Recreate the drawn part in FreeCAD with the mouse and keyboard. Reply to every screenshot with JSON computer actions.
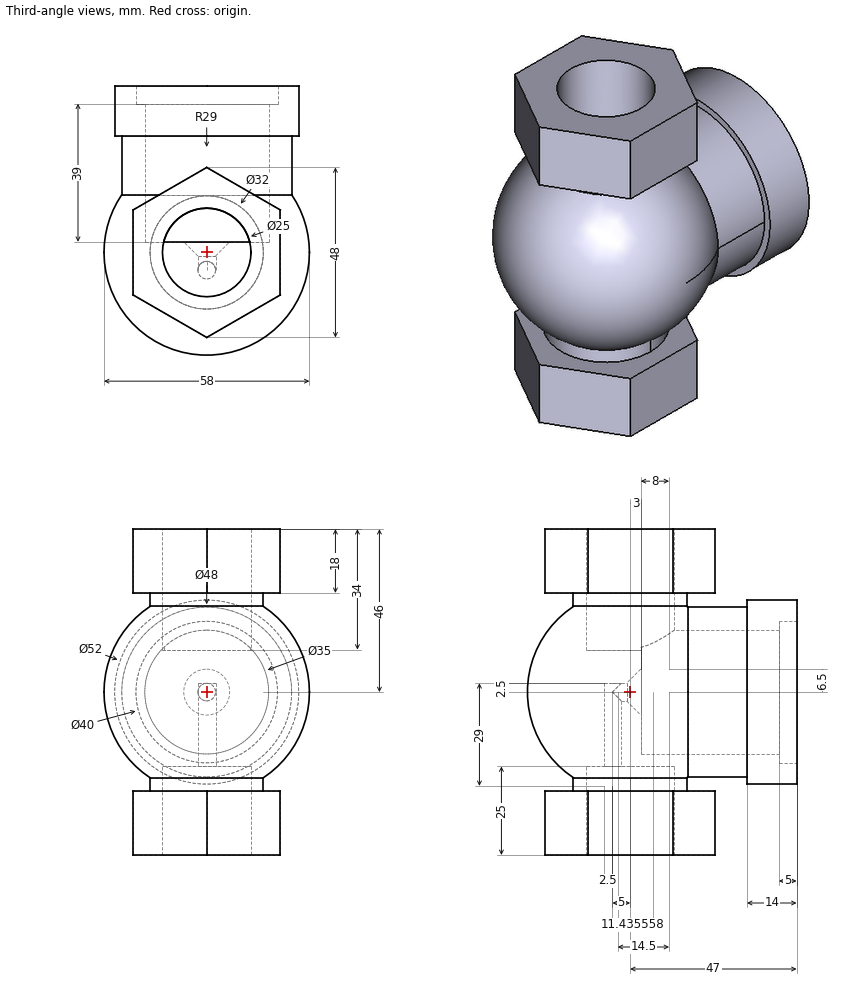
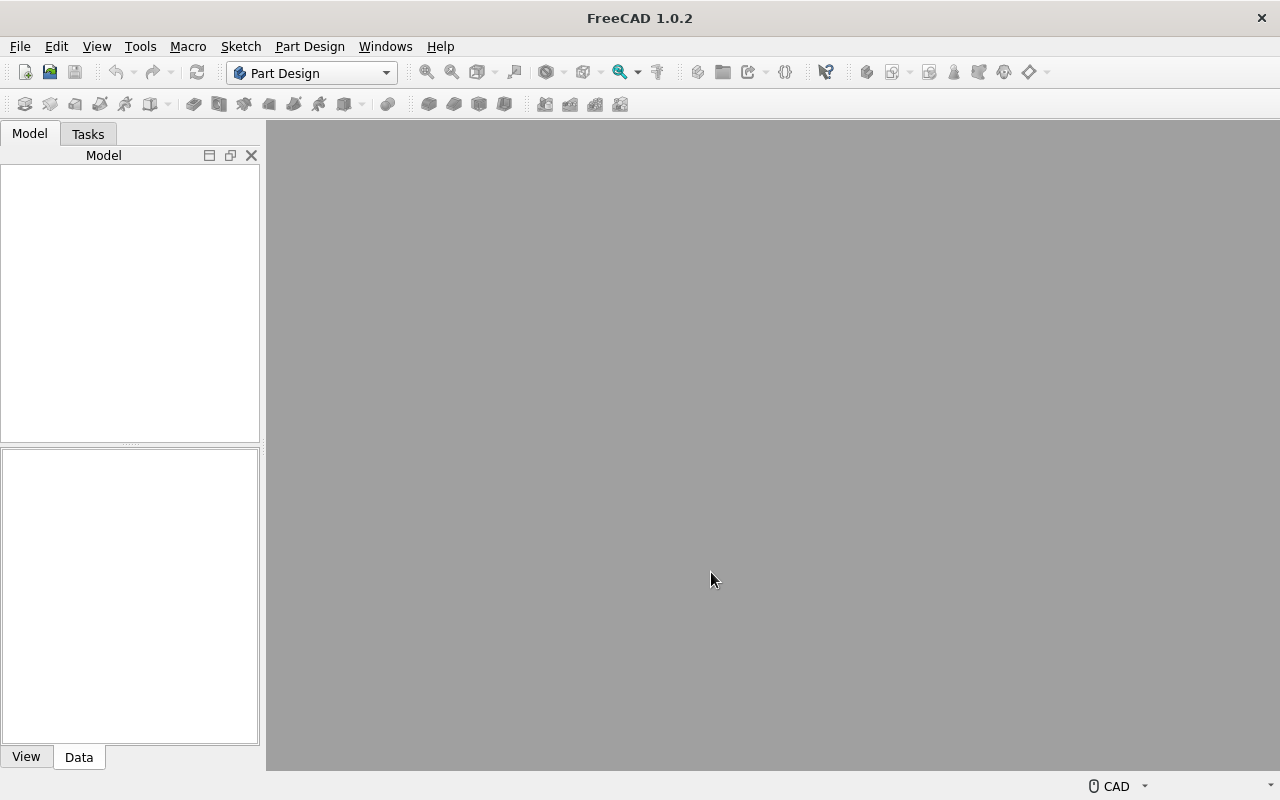
{"action": "left_click", "coordinate": [25, 72]}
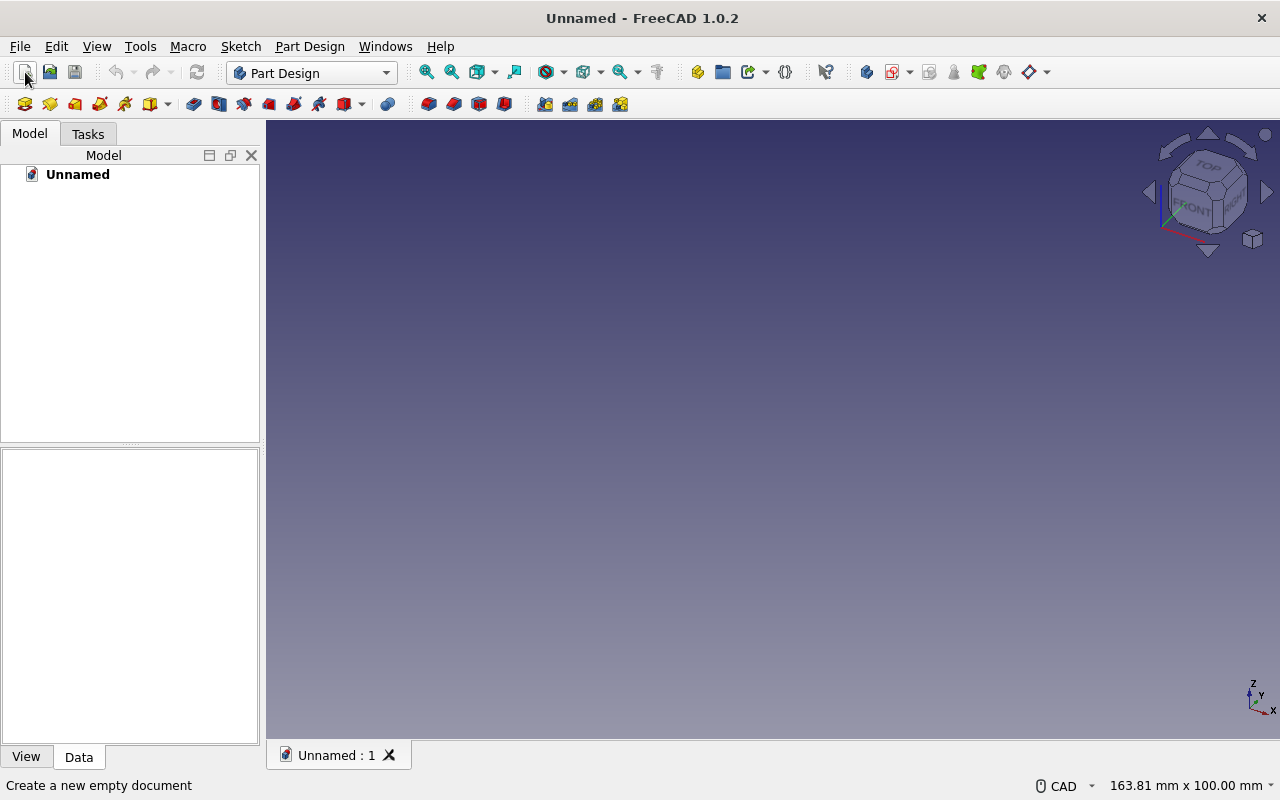
{"action": "left_click", "coordinate": [892, 72]}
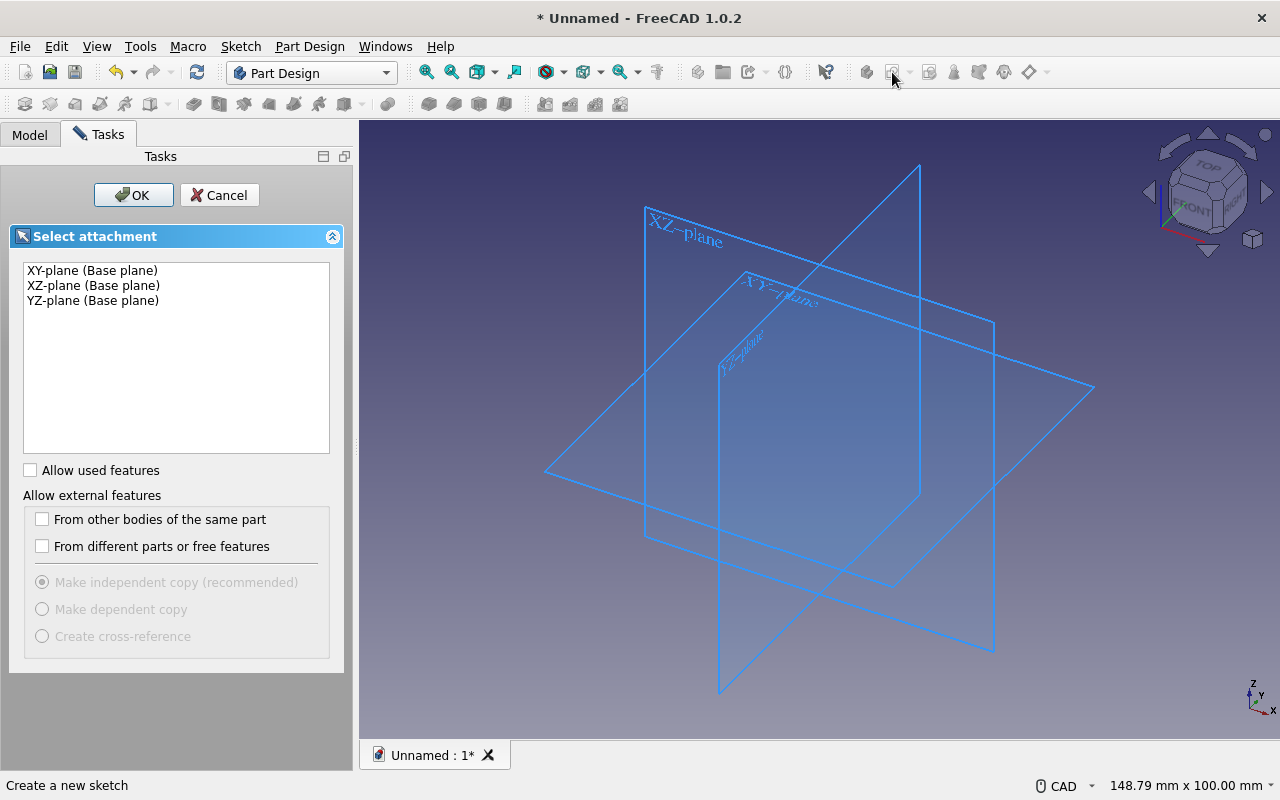
{"action": "left_click", "coordinate": [84, 270]}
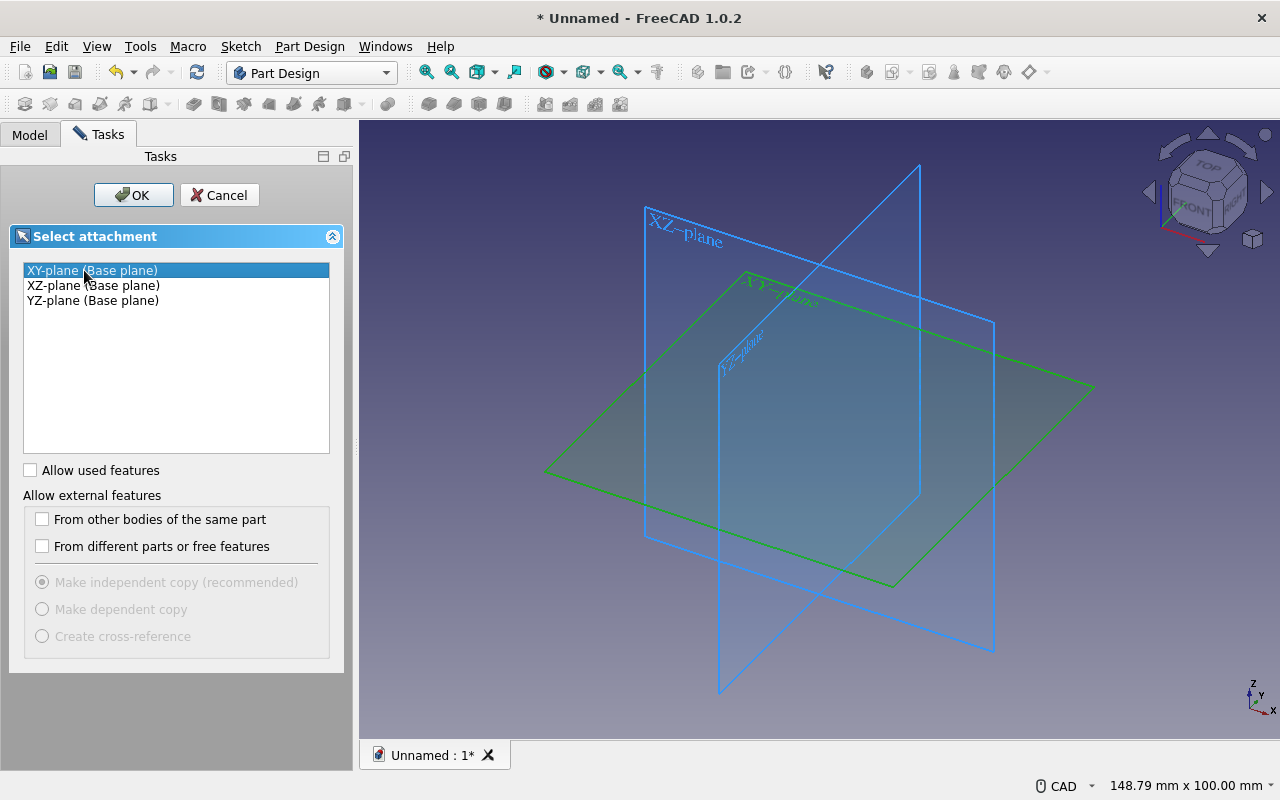
{"action": "left_click", "coordinate": [134, 195]}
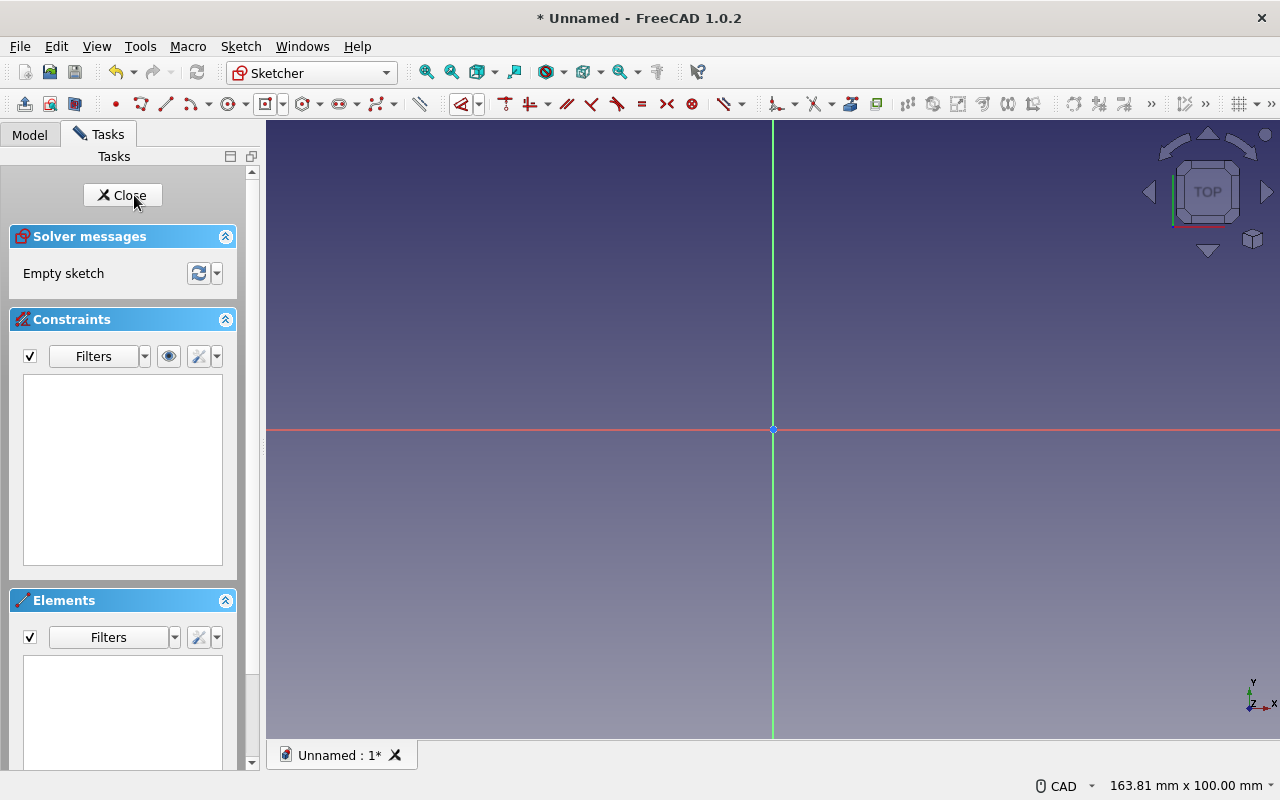
{"action": "scroll", "coordinate": [912, 157], "scroll_direction": "up", "scroll_amount": 2}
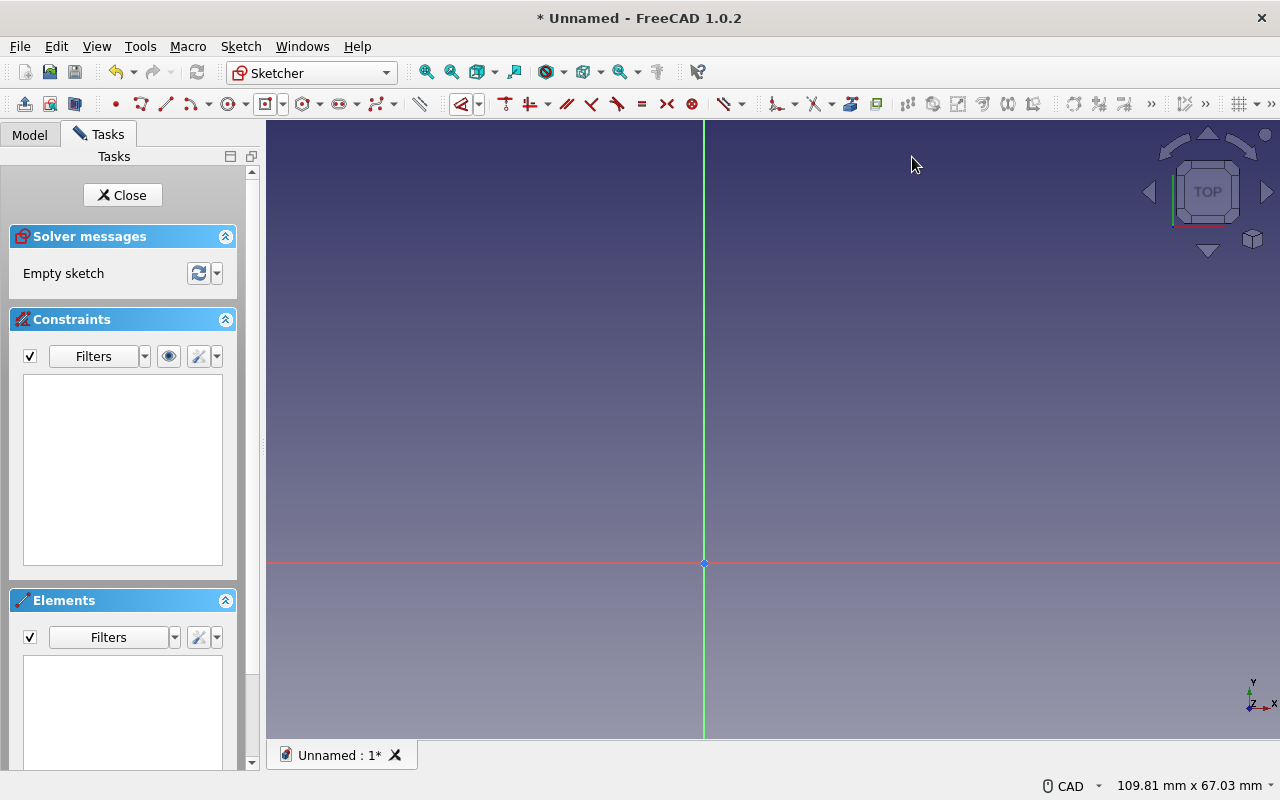
{"action": "left_click", "coordinate": [166, 104]}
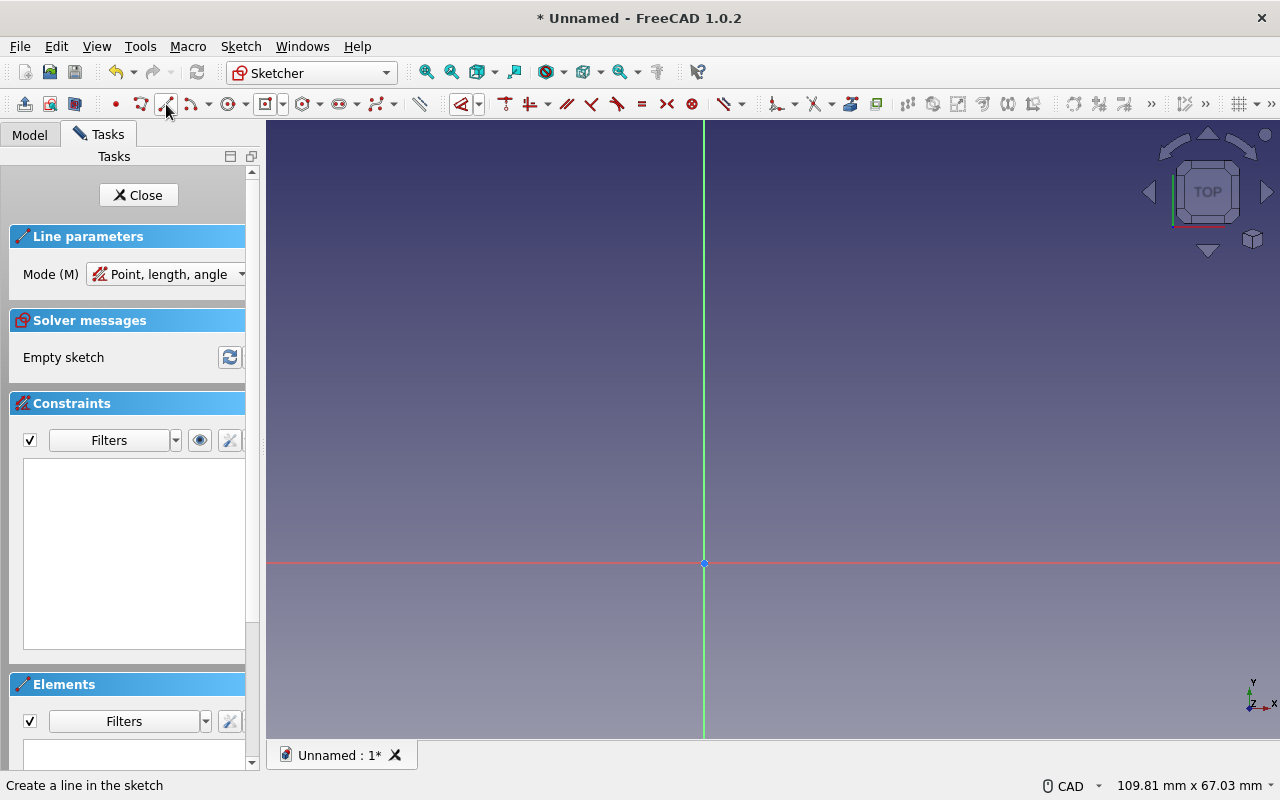
{"action": "left_click", "coordinate": [437, 563]}
{"action": "left_click", "coordinate": [972, 554]}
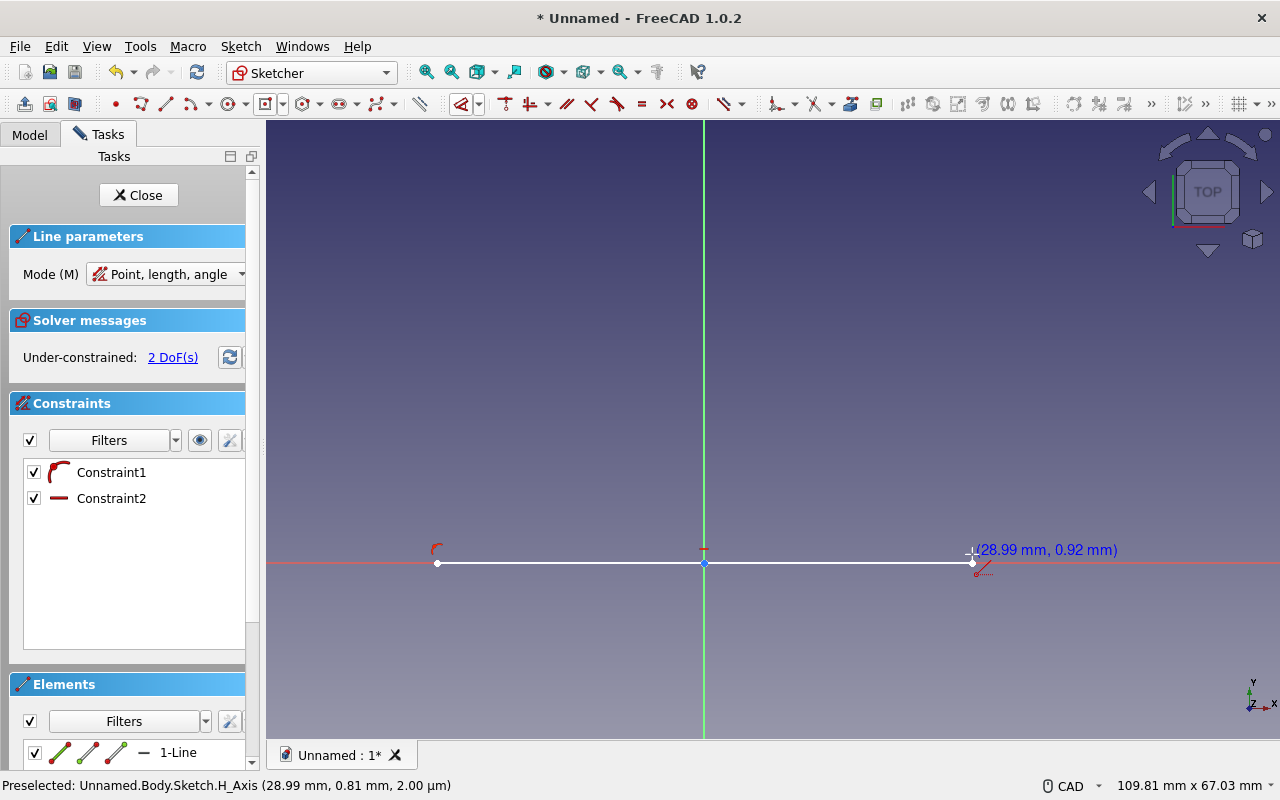
{"action": "left_click", "coordinate": [208, 104]}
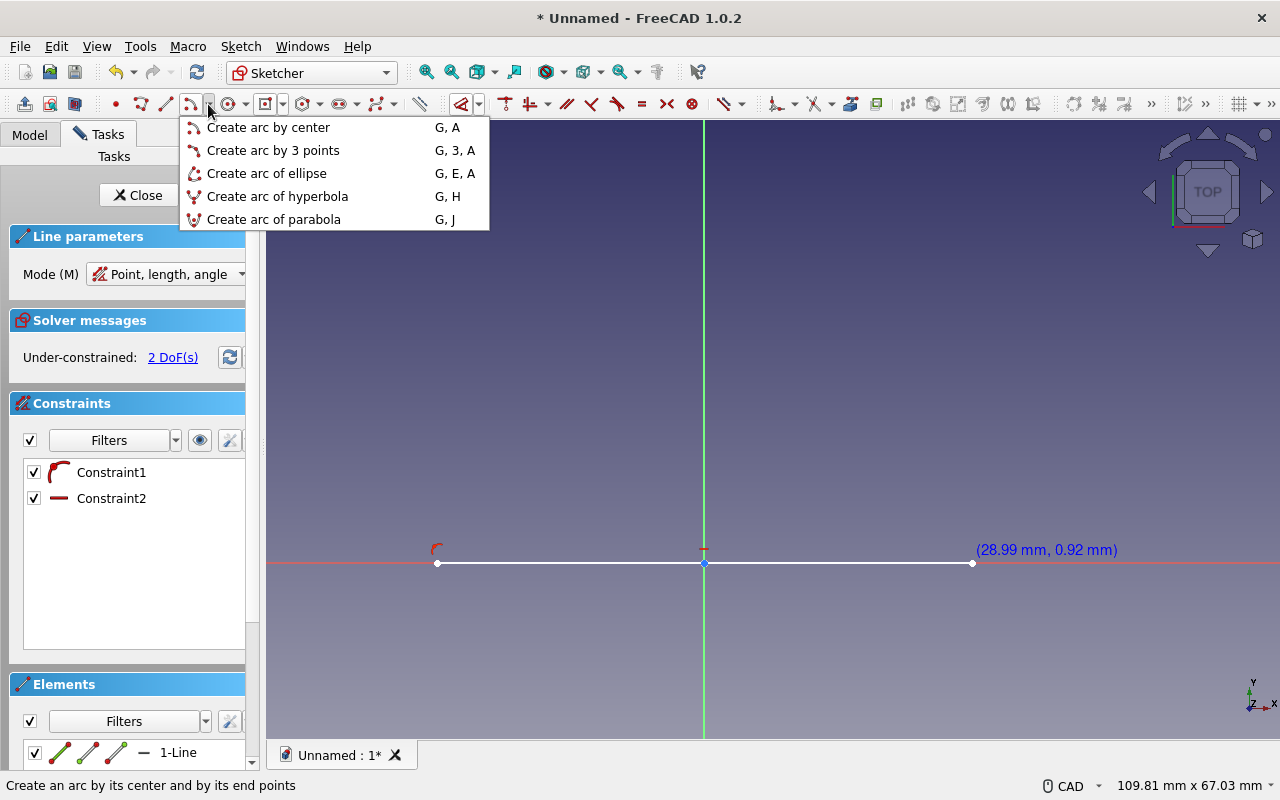
{"action": "left_click", "coordinate": [334, 150]}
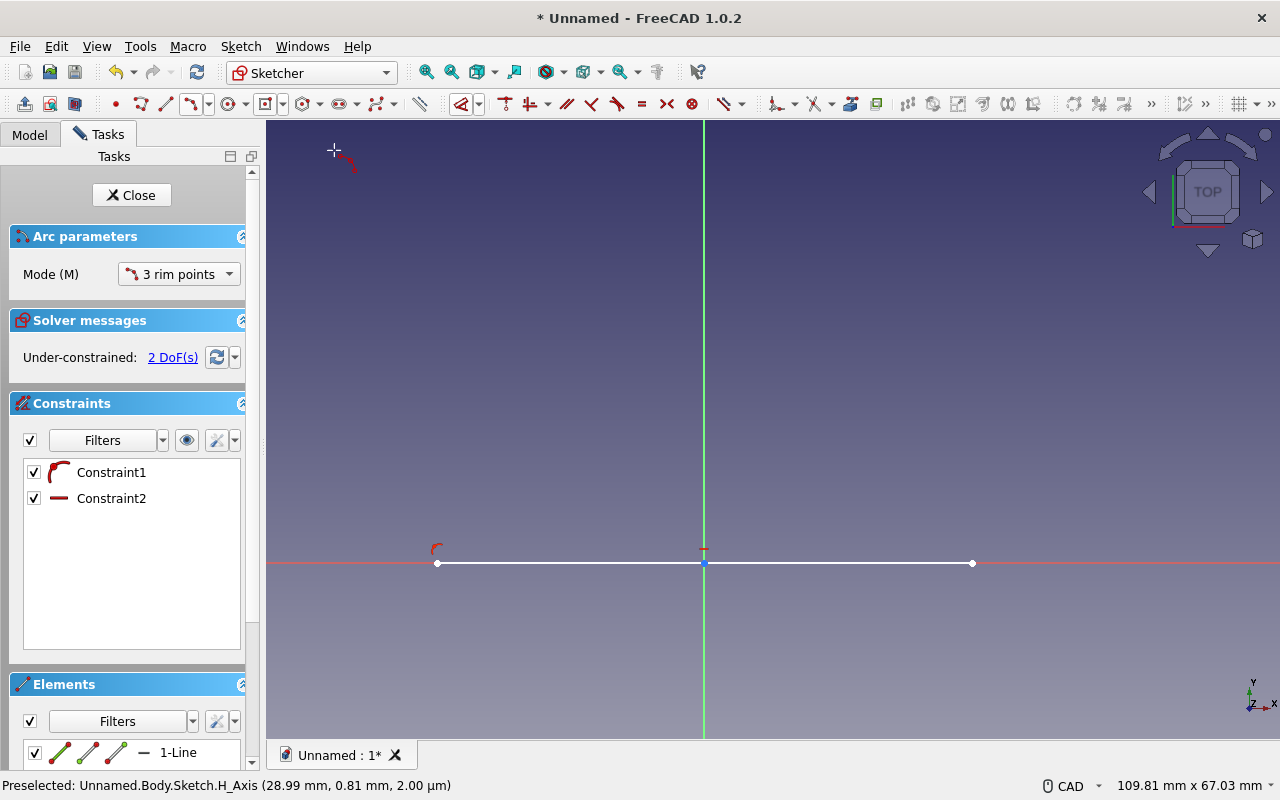
{"action": "left_click", "coordinate": [972, 554]}
{"action": "left_click", "coordinate": [437, 563]}
{"action": "left_click", "coordinate": [787, 309]}
{"action": "key", "text": "Escape"}